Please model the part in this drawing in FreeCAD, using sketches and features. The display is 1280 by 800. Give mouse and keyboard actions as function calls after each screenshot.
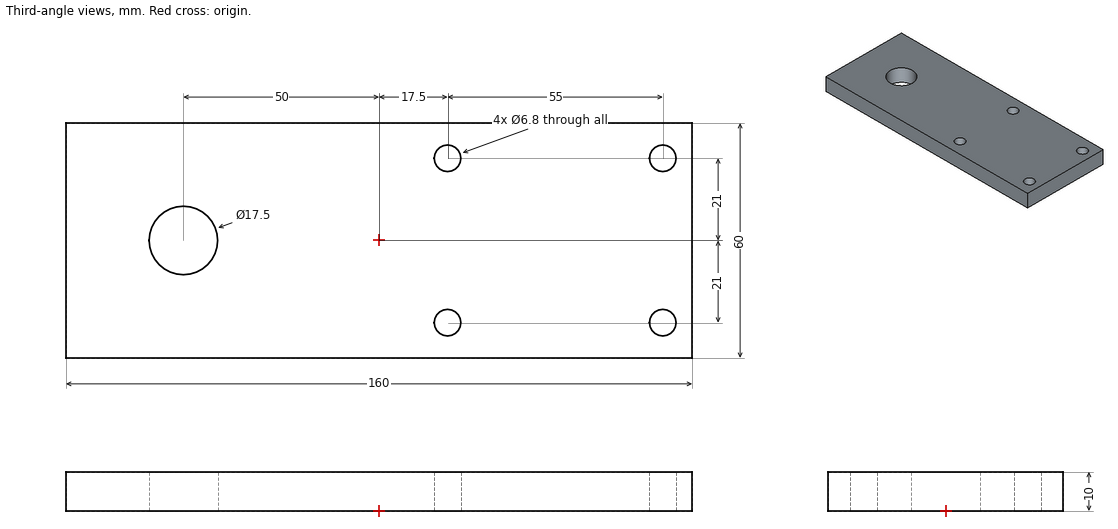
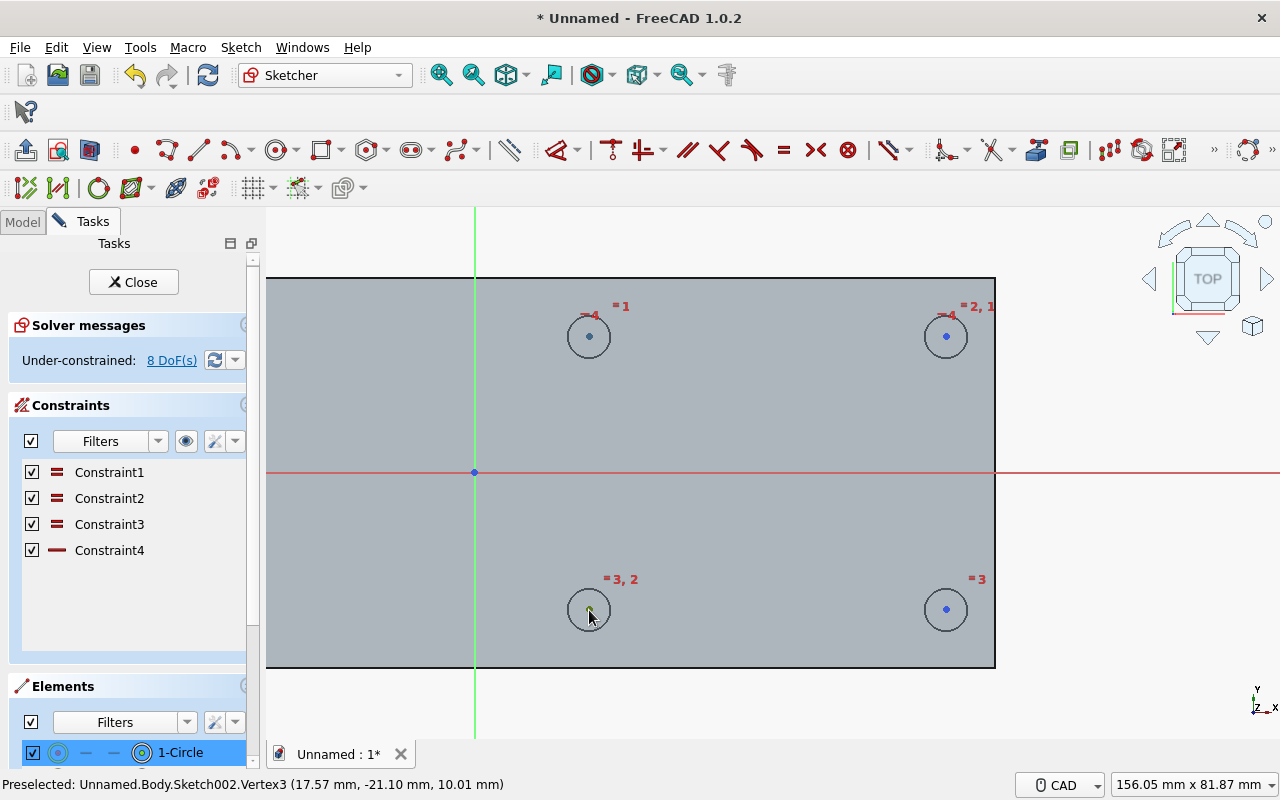
key(v)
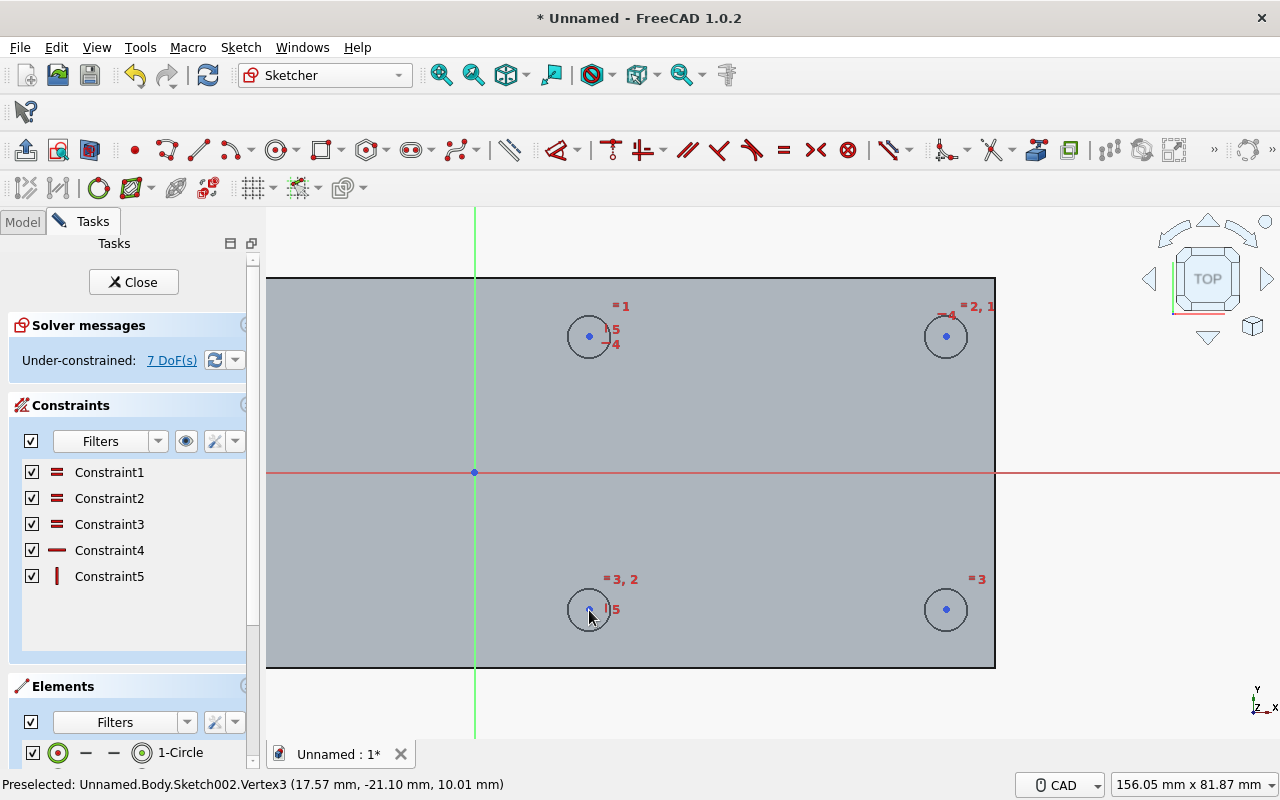
click(946, 337)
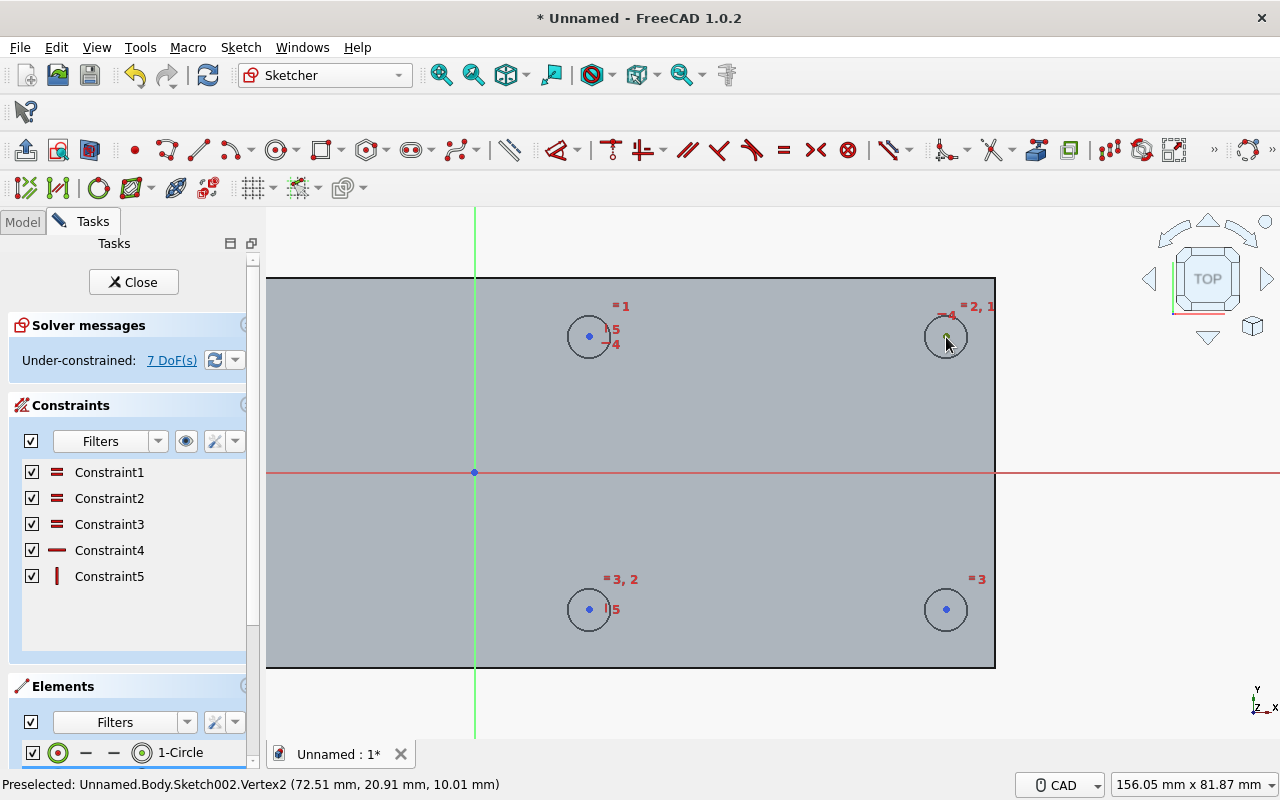
click(946, 610)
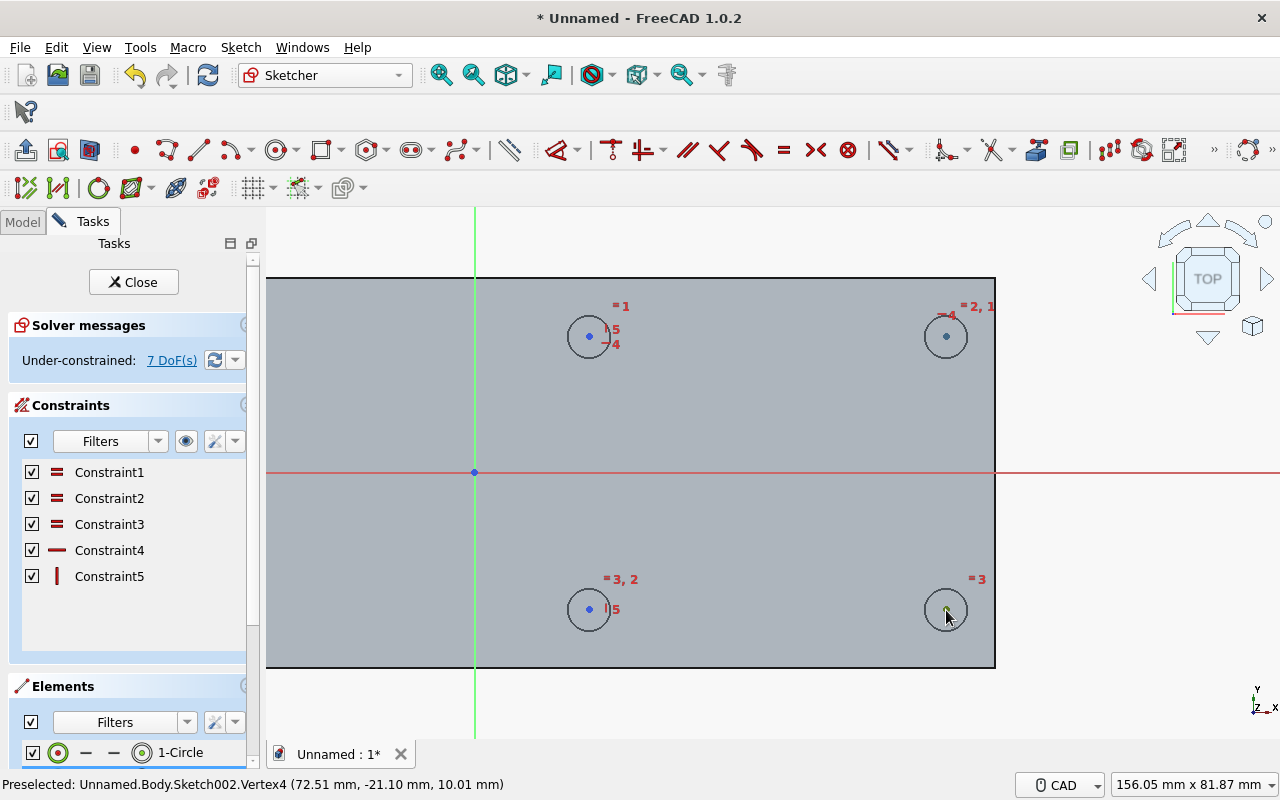
key(v)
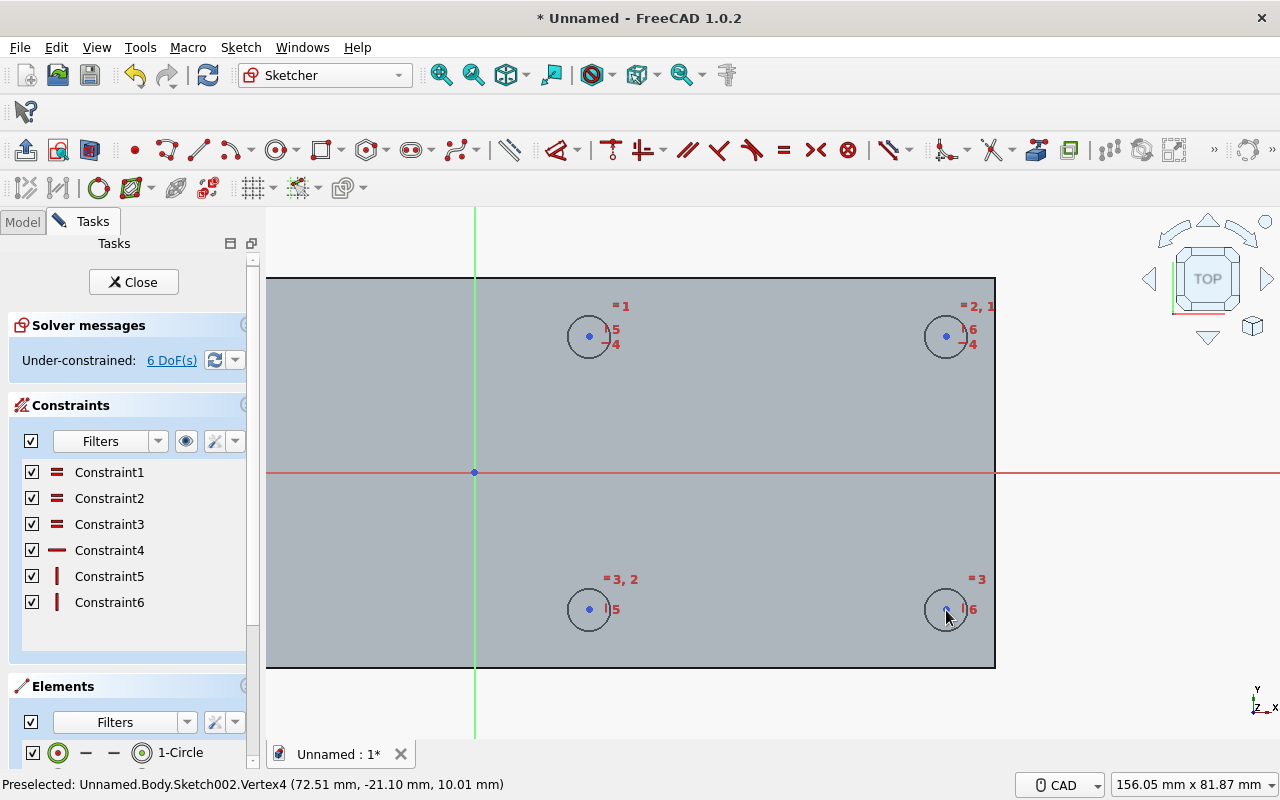
click(589, 610)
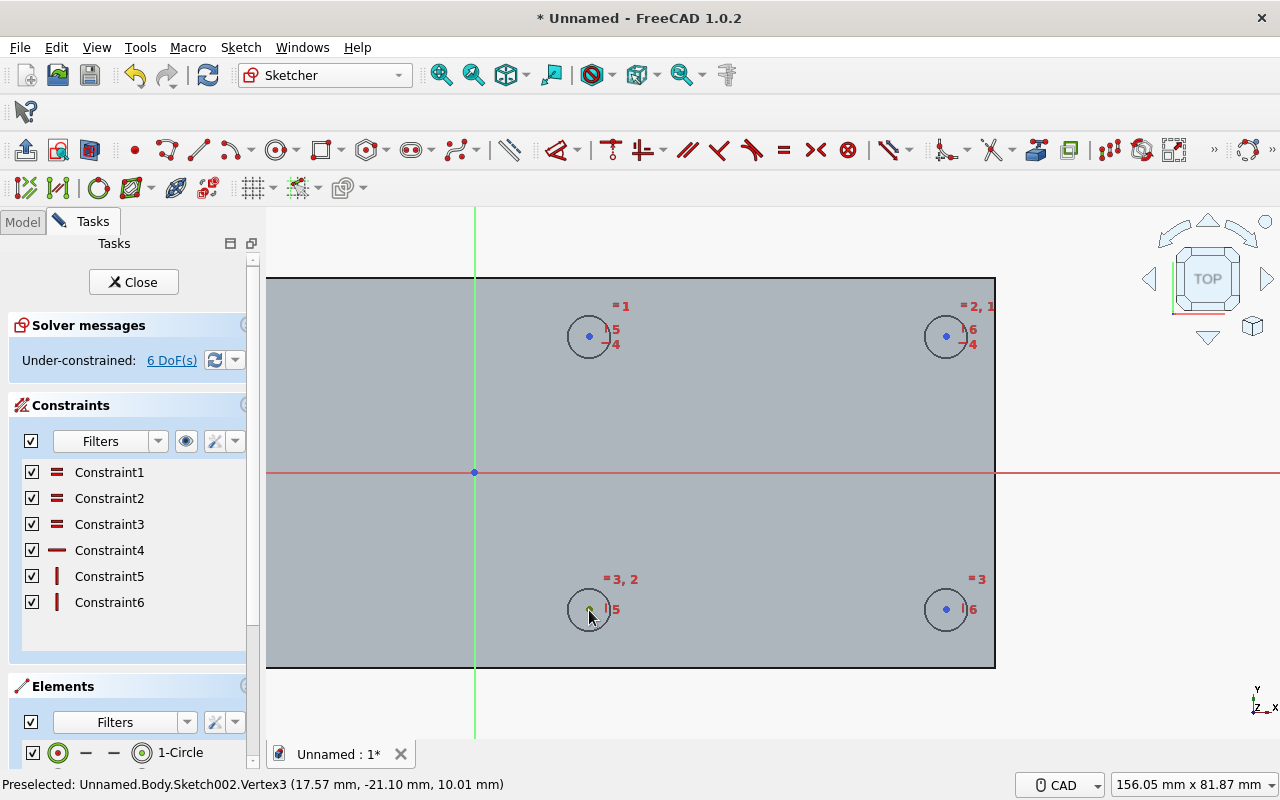
click(946, 610)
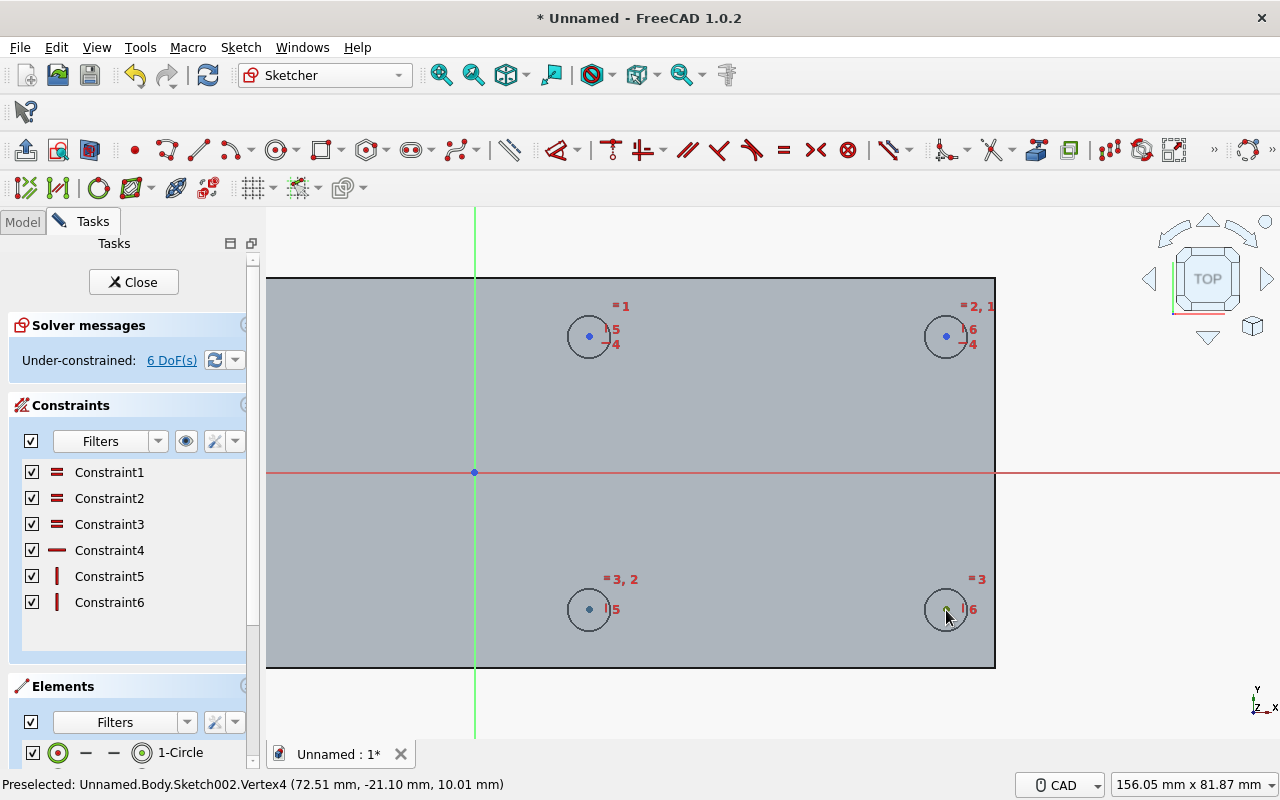
key(h)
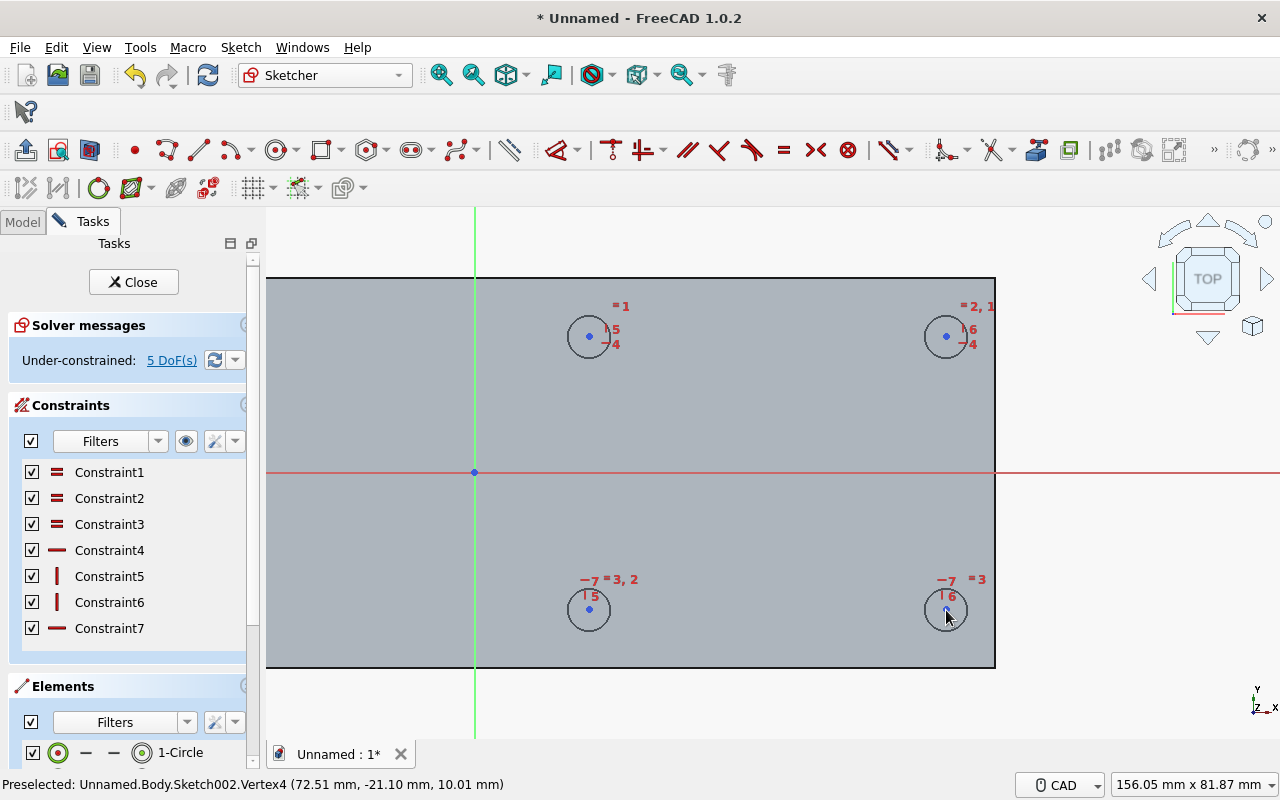
key(d)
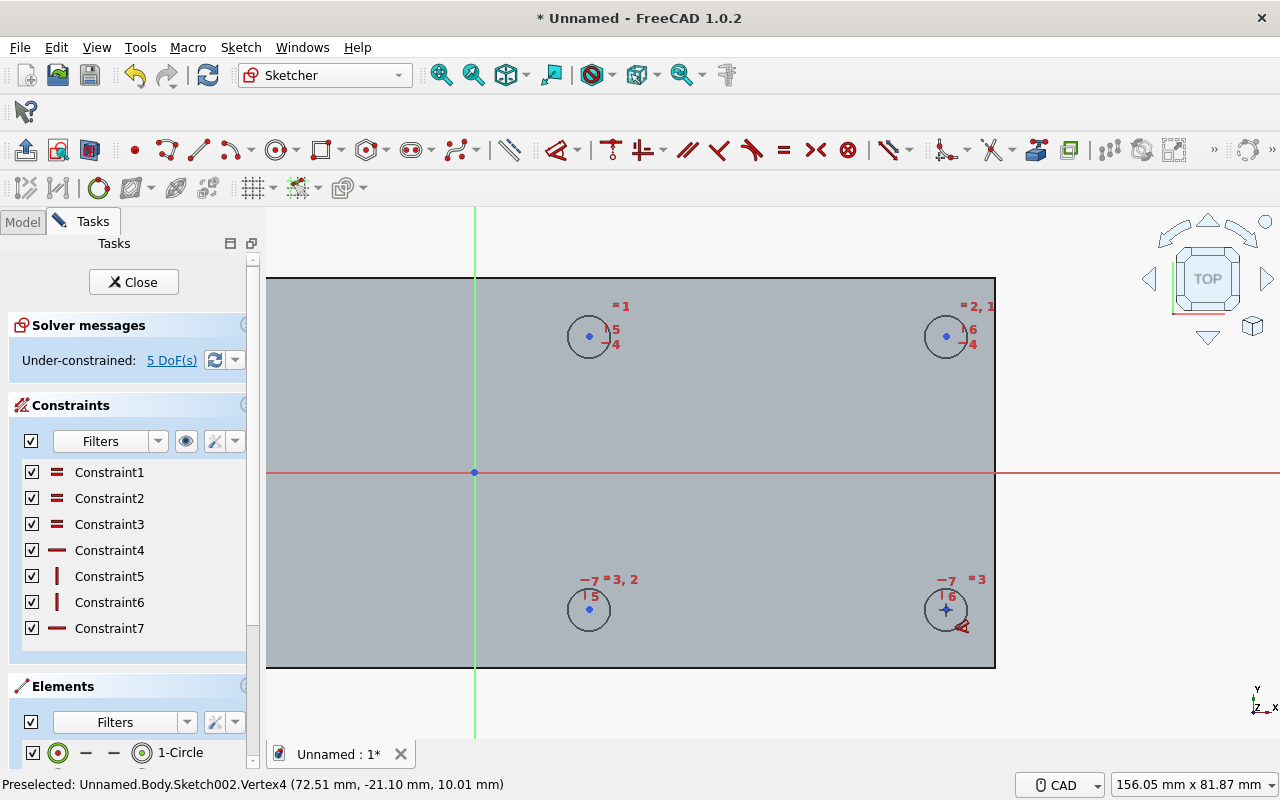
click(604, 322)
click(627, 299)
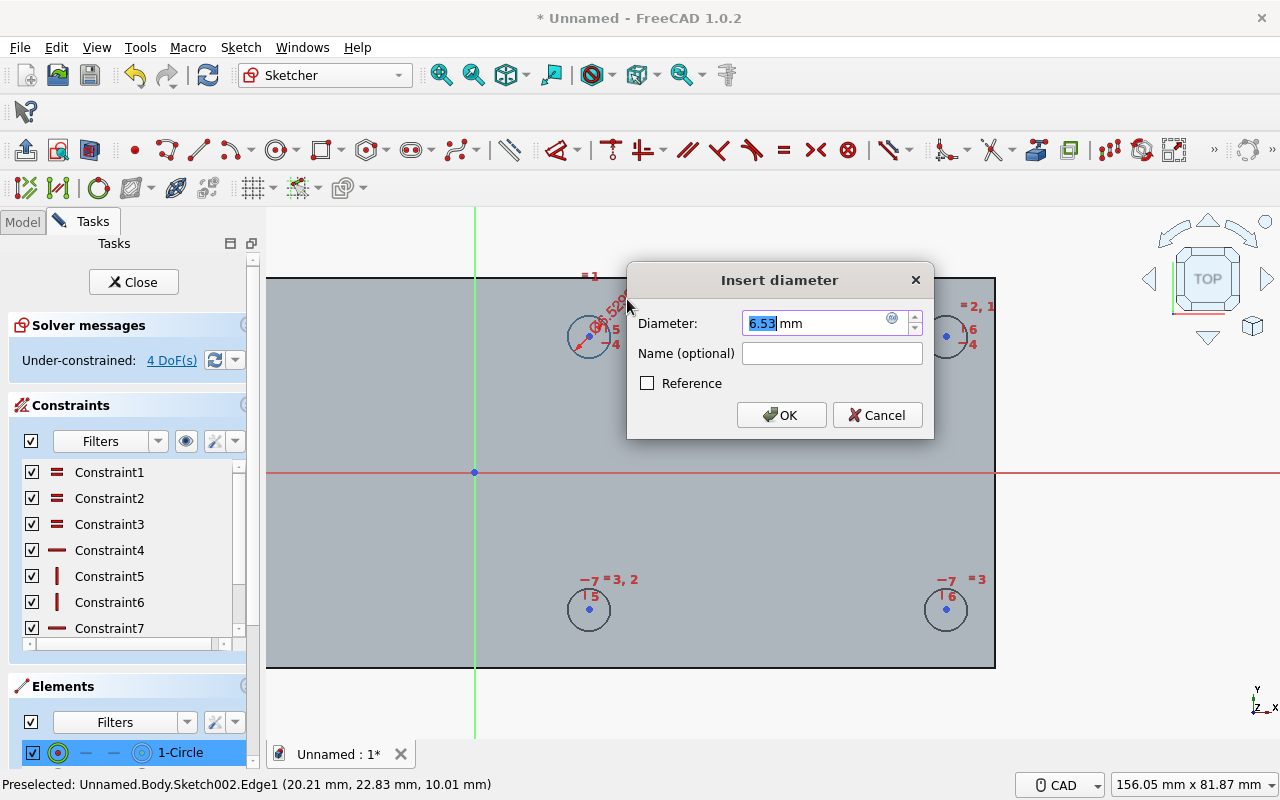
text(6.8)
key(Return)